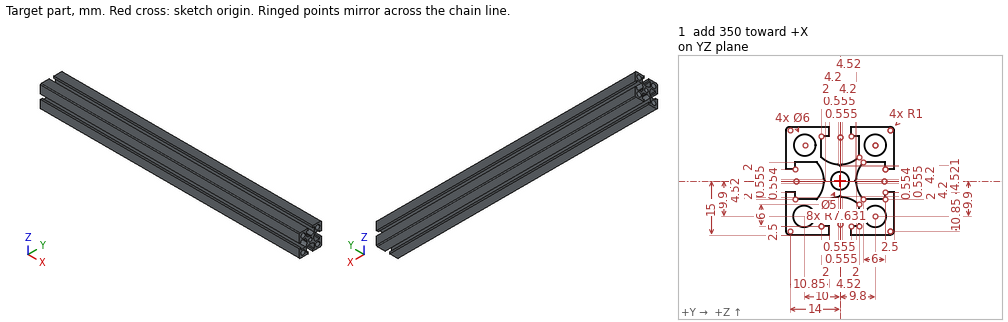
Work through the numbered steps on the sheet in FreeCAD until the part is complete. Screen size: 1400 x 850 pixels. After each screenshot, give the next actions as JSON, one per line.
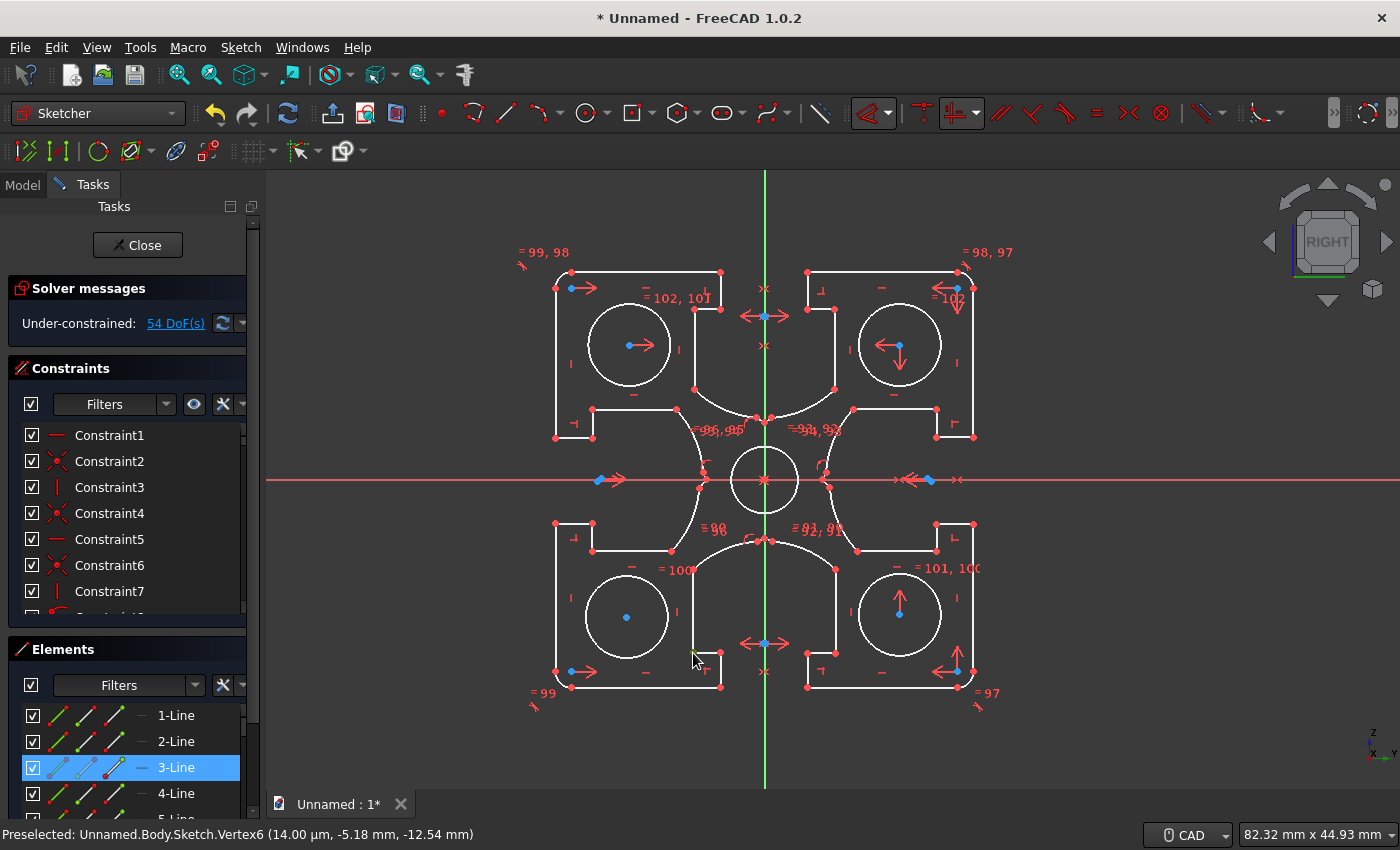
{"action": "left_click", "coordinate": [836, 653]}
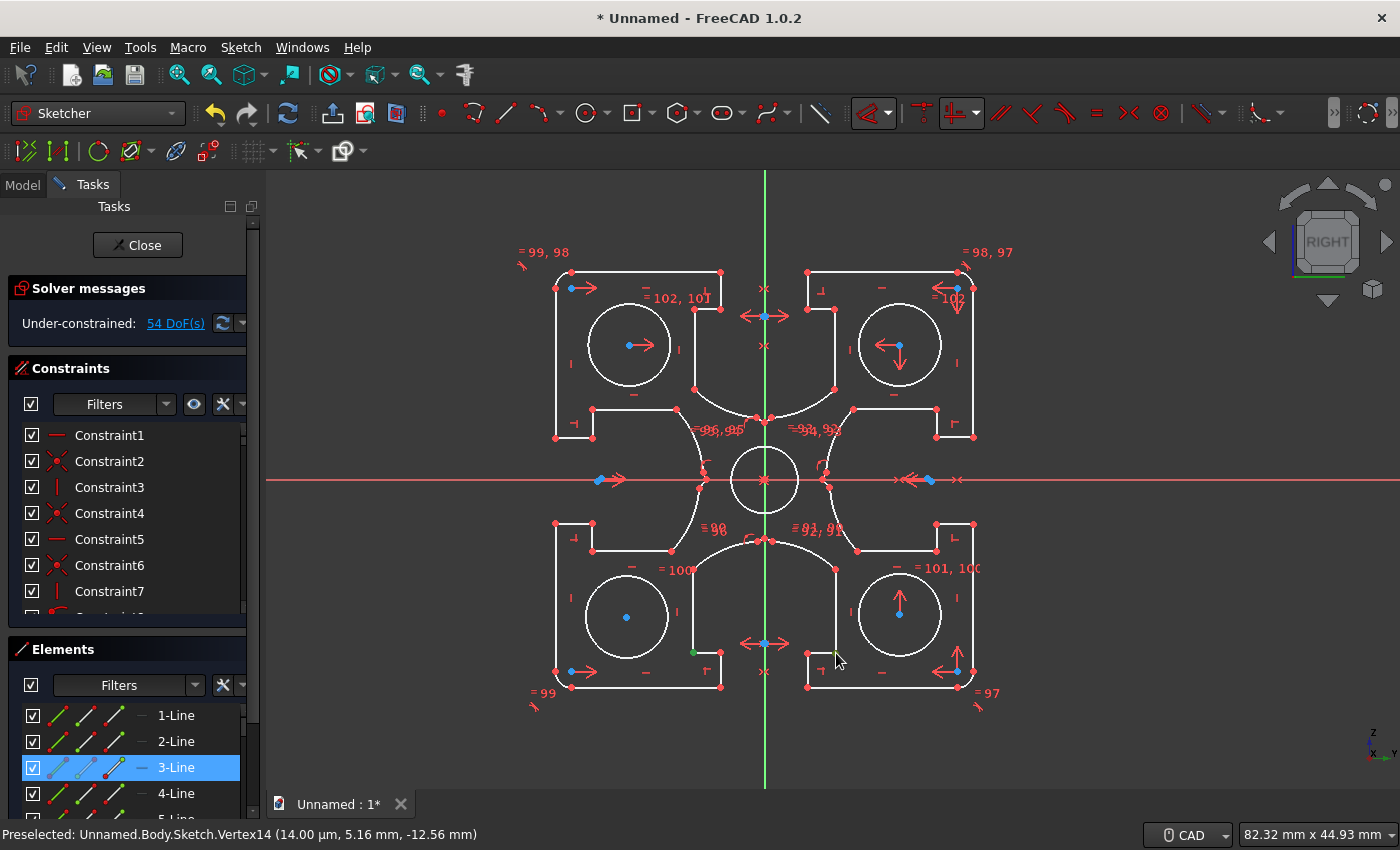
{"action": "left_click", "coordinate": [765, 721]}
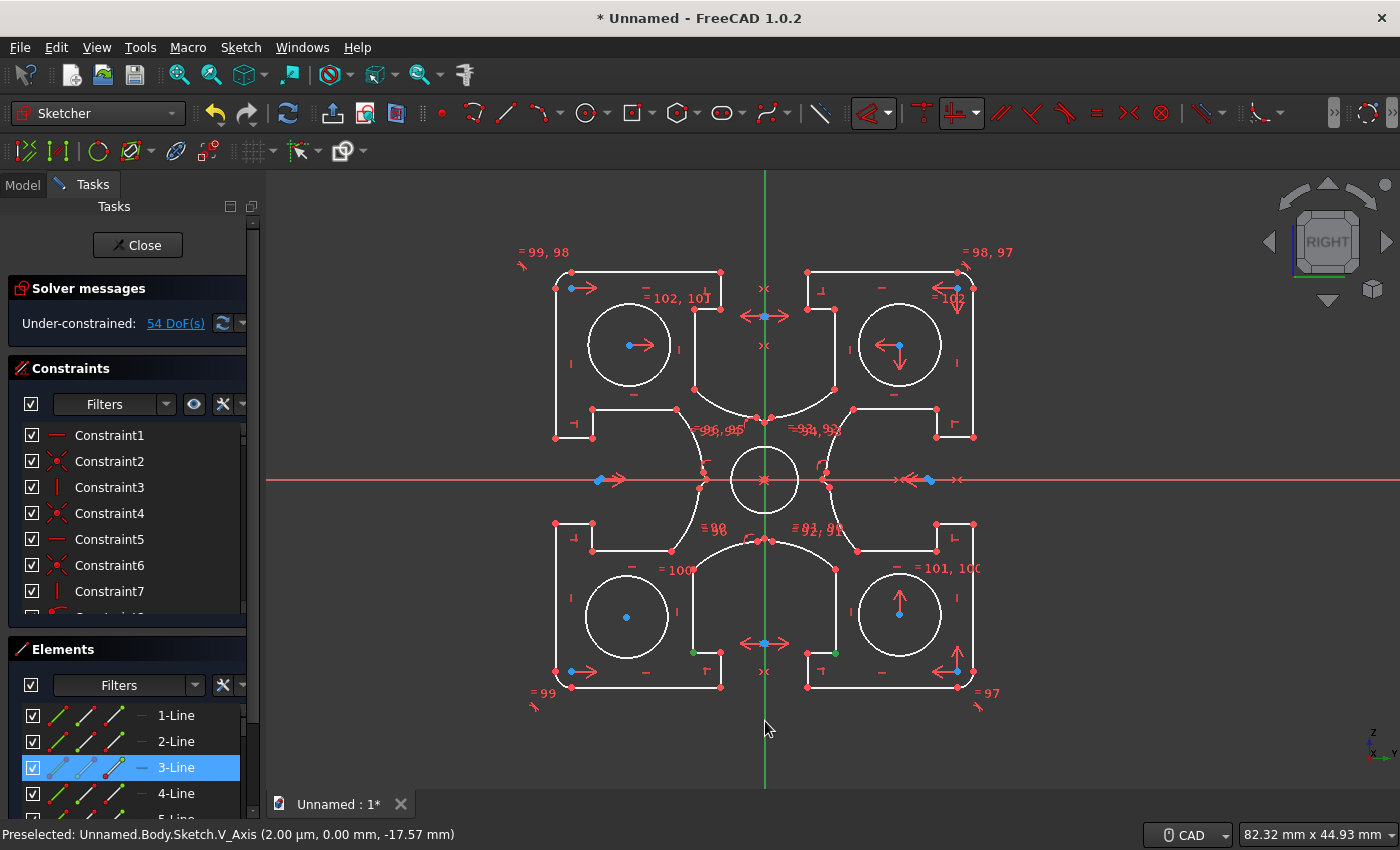
{"action": "left_click", "coordinate": [1130, 114]}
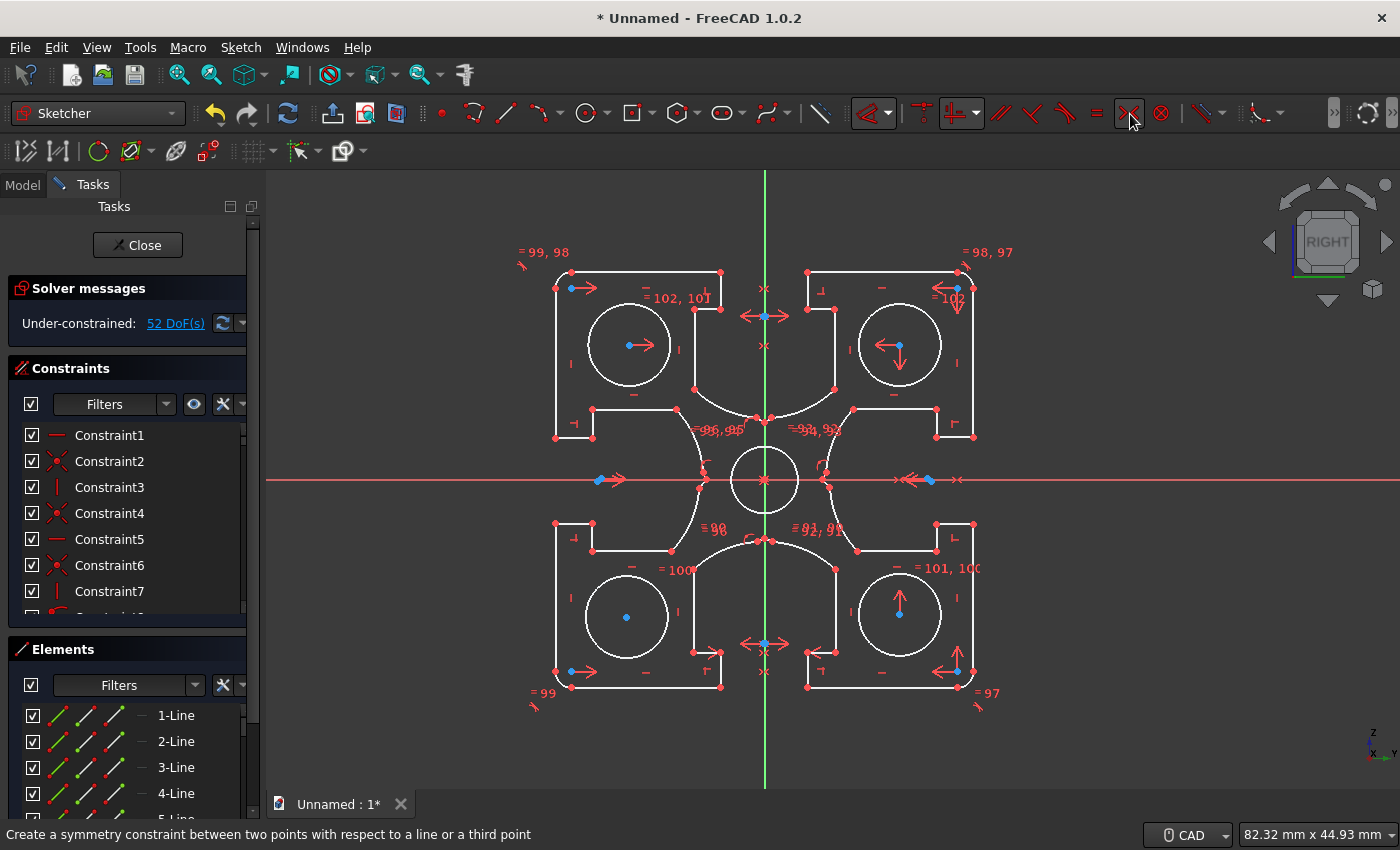
{"action": "left_click", "coordinate": [858, 551]}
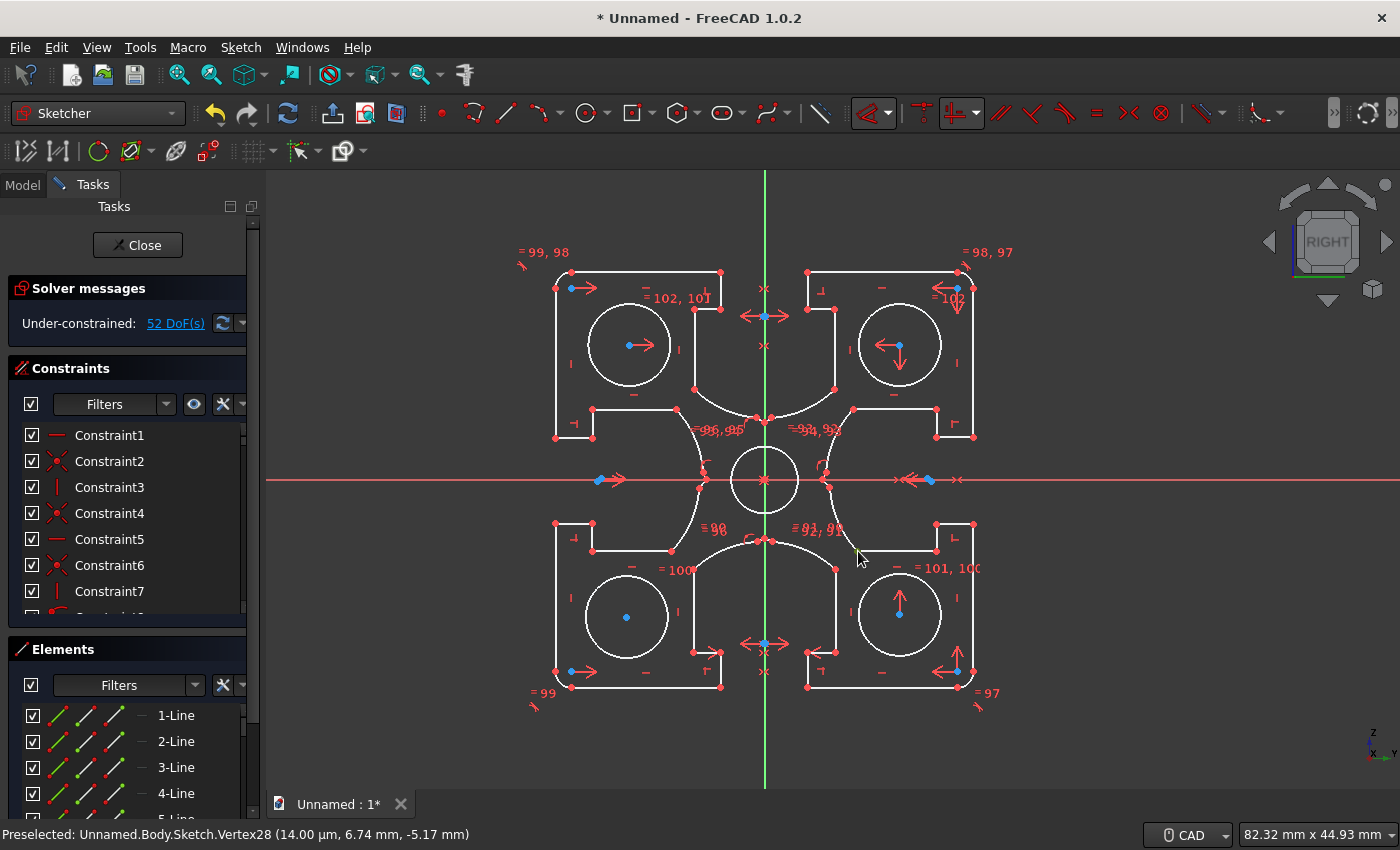
{"action": "left_click", "coordinate": [853, 409]}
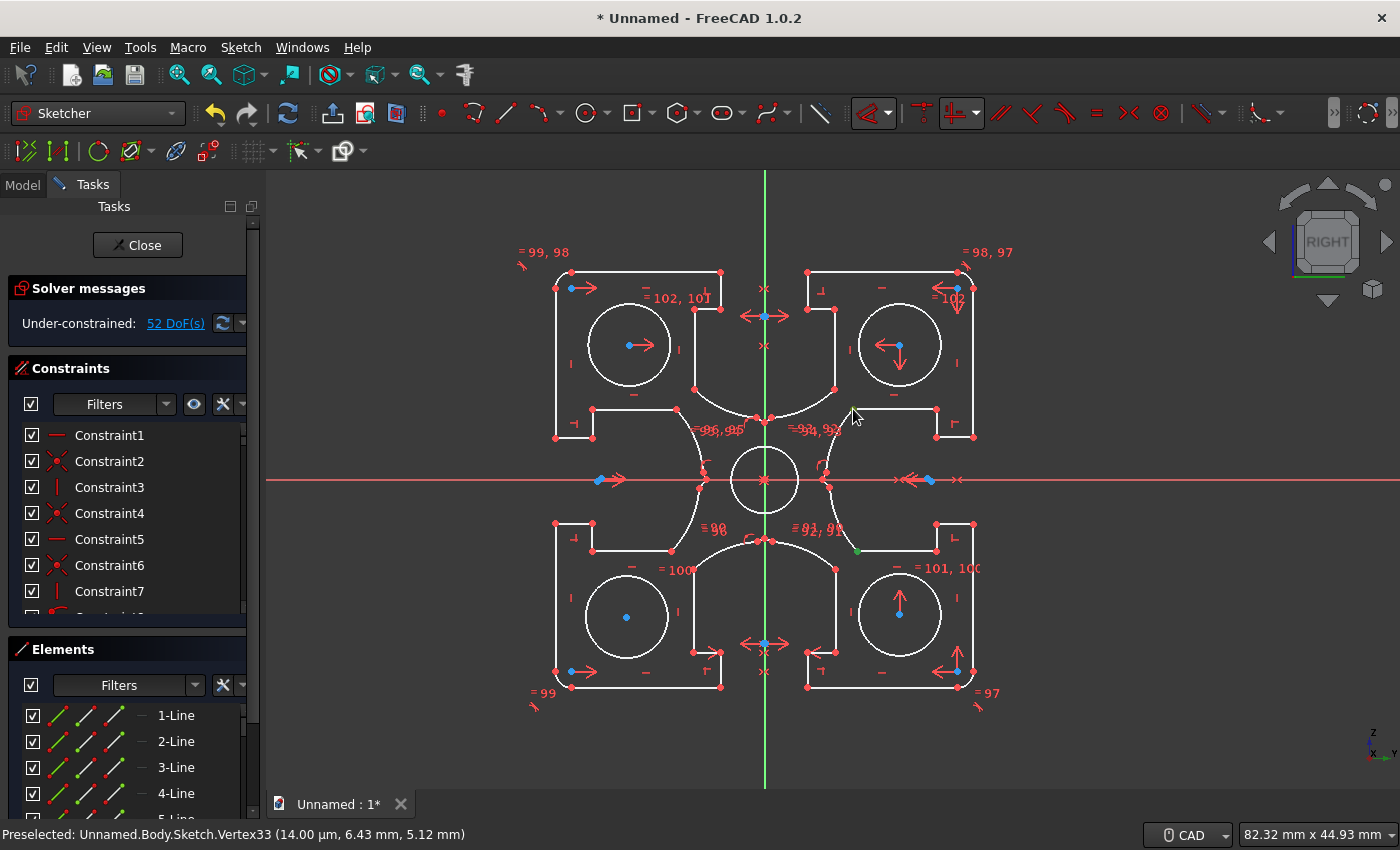
{"action": "left_click", "coordinate": [361, 480]}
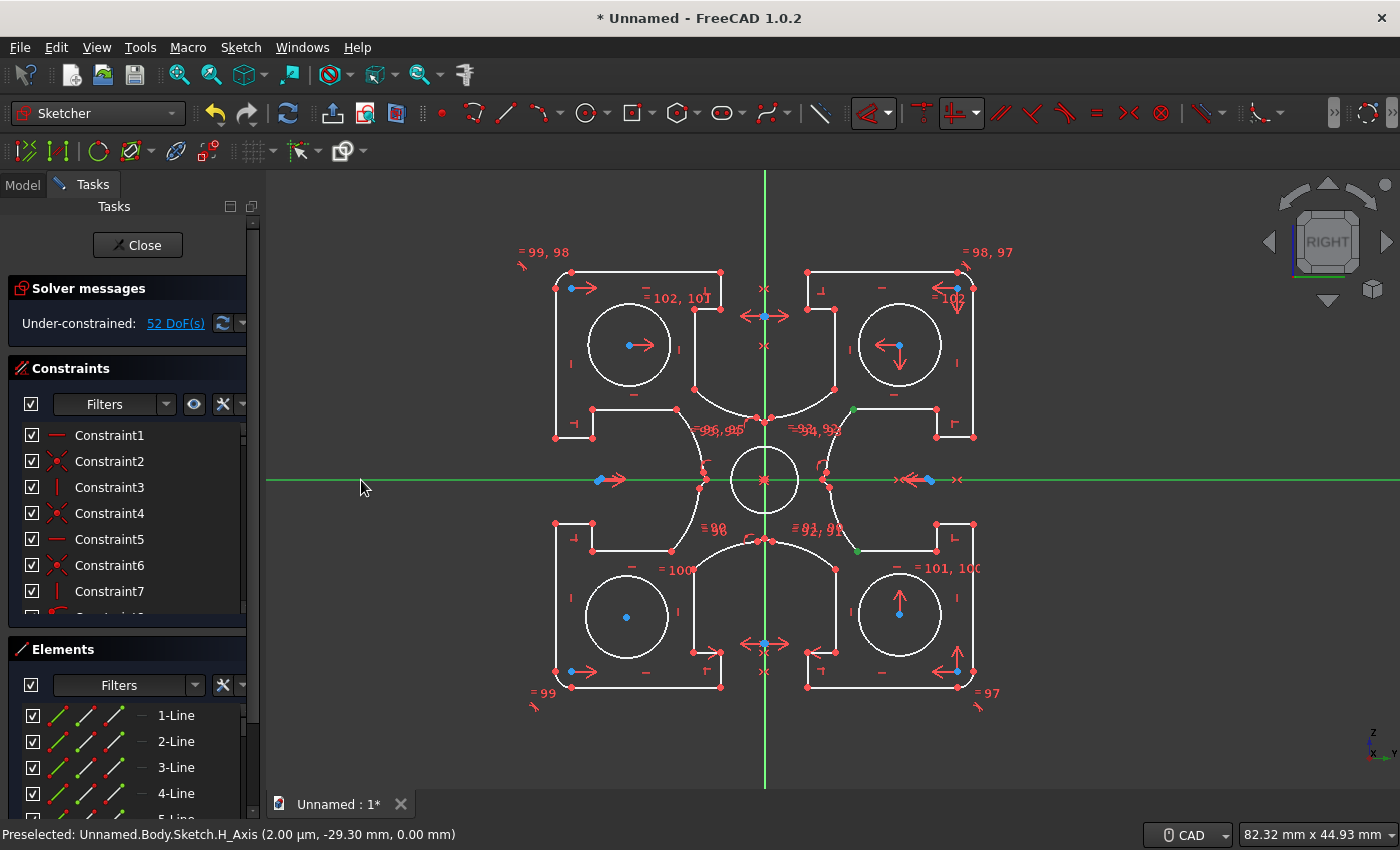
{"action": "left_click", "coordinate": [1130, 114]}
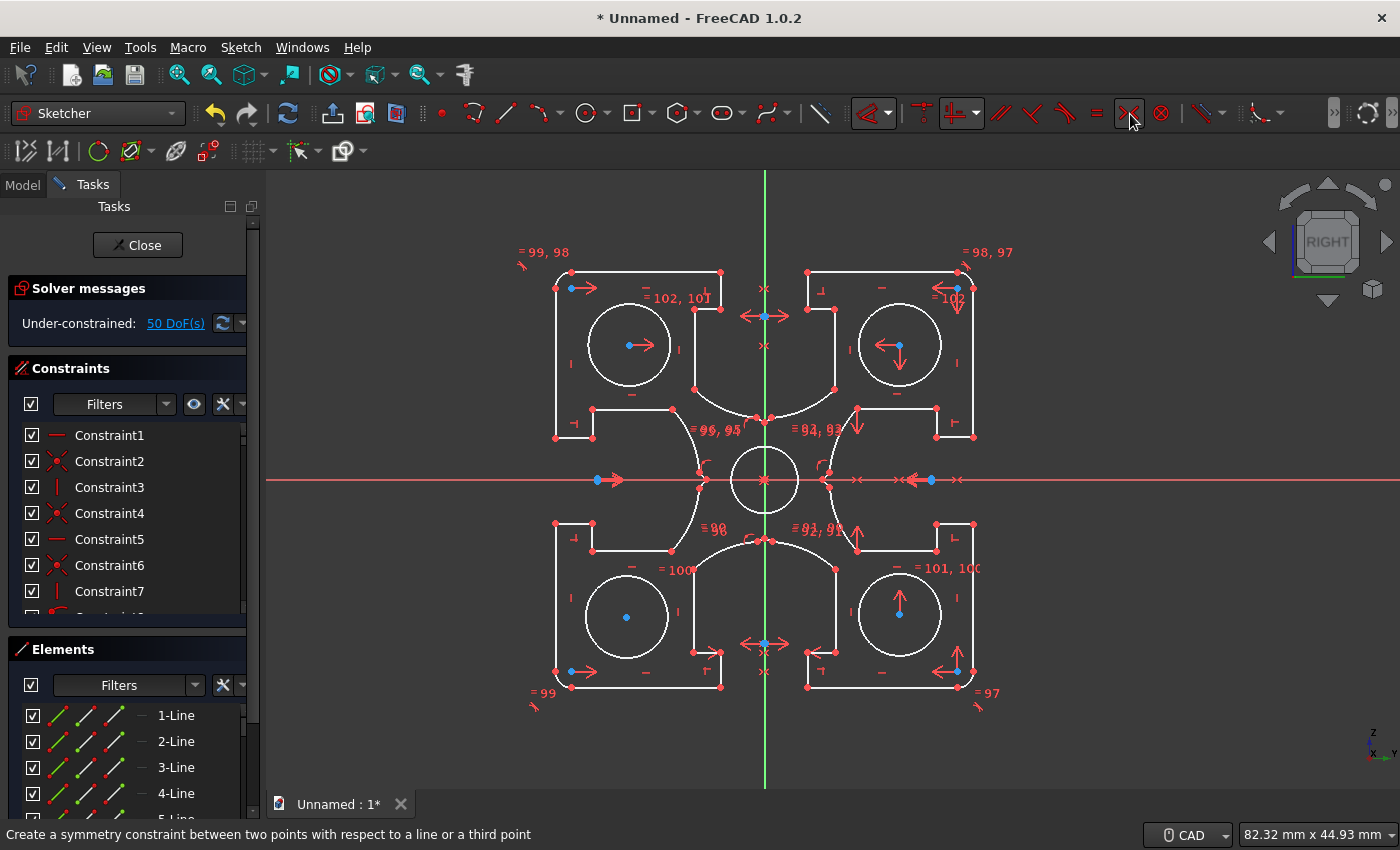
{"action": "left_click", "coordinate": [937, 524]}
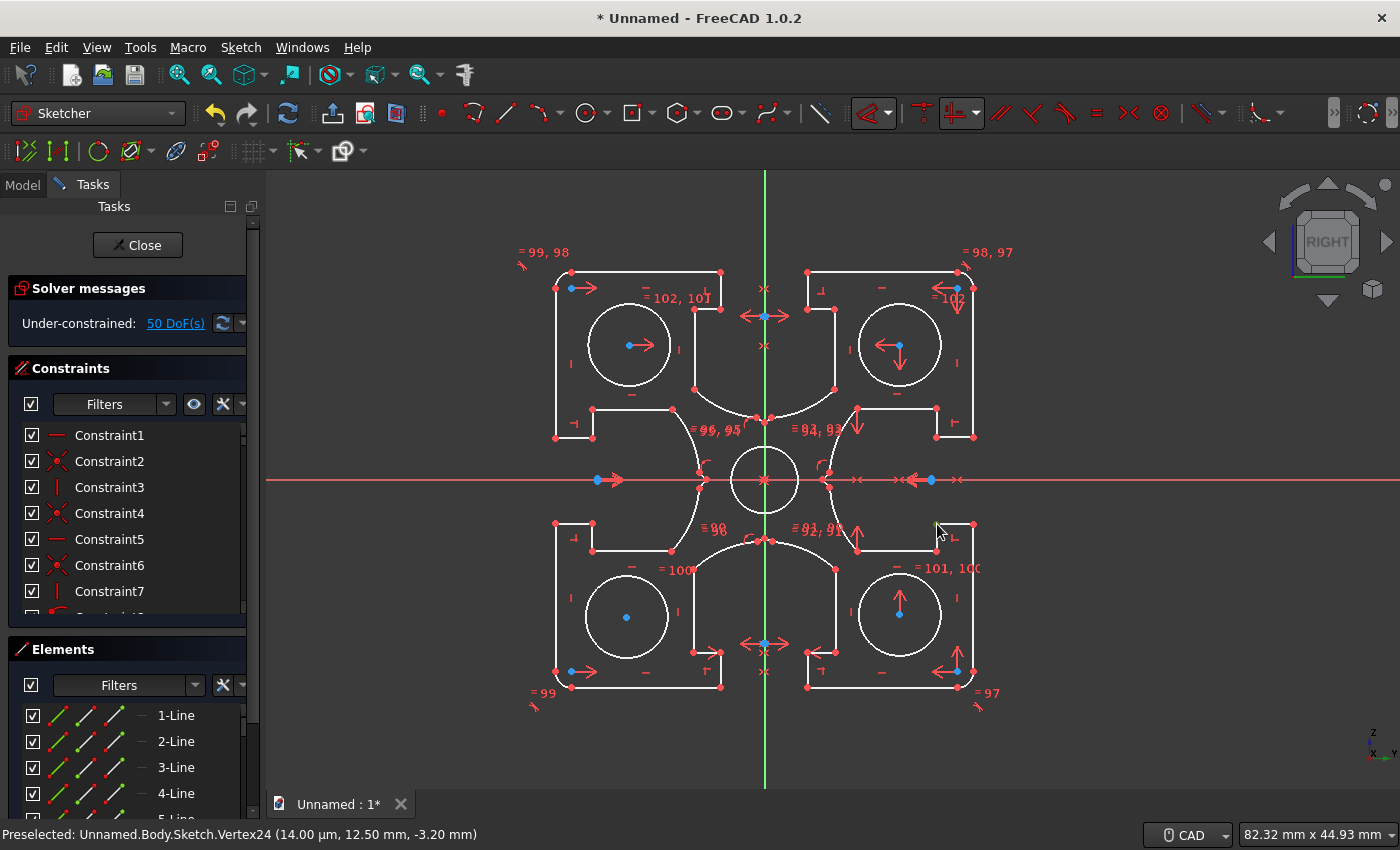
{"action": "left_click", "coordinate": [937, 437]}